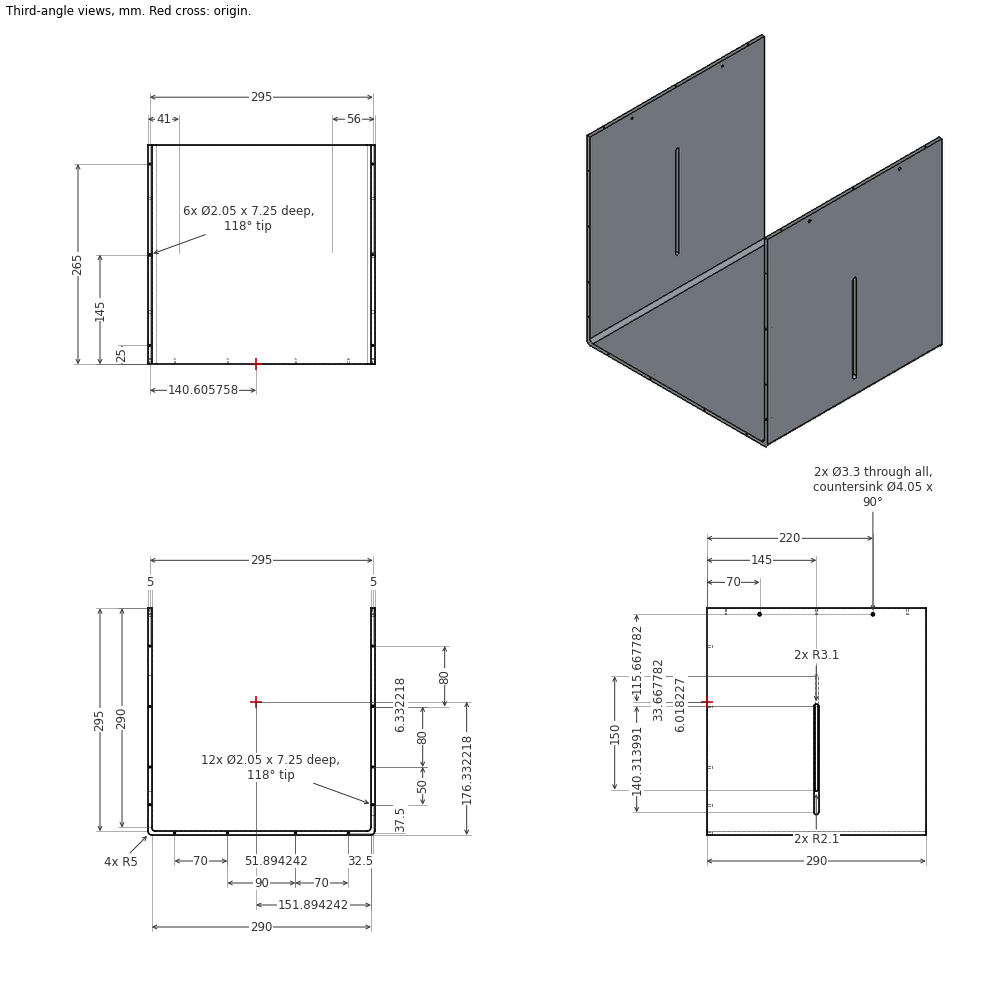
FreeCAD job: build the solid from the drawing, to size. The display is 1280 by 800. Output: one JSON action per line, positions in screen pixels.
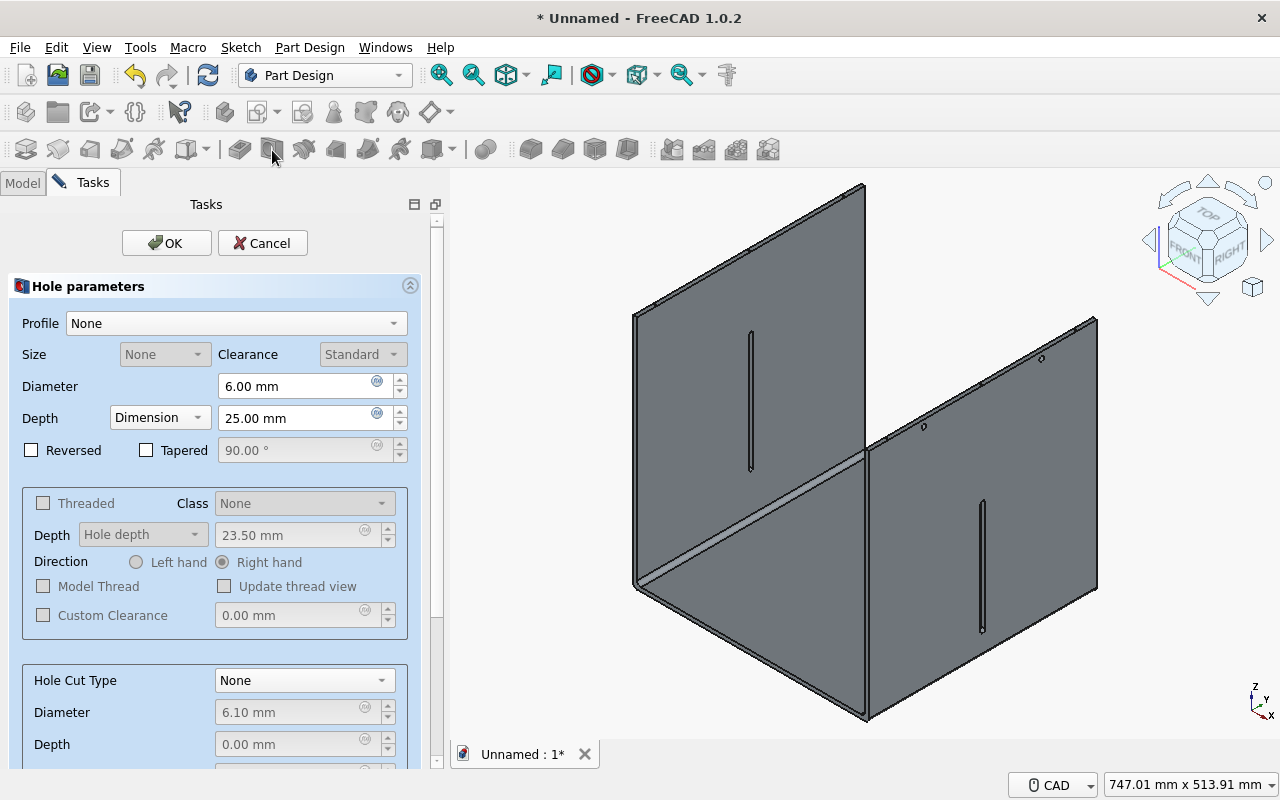
{"action": "triple_click", "coordinate": [305, 386]}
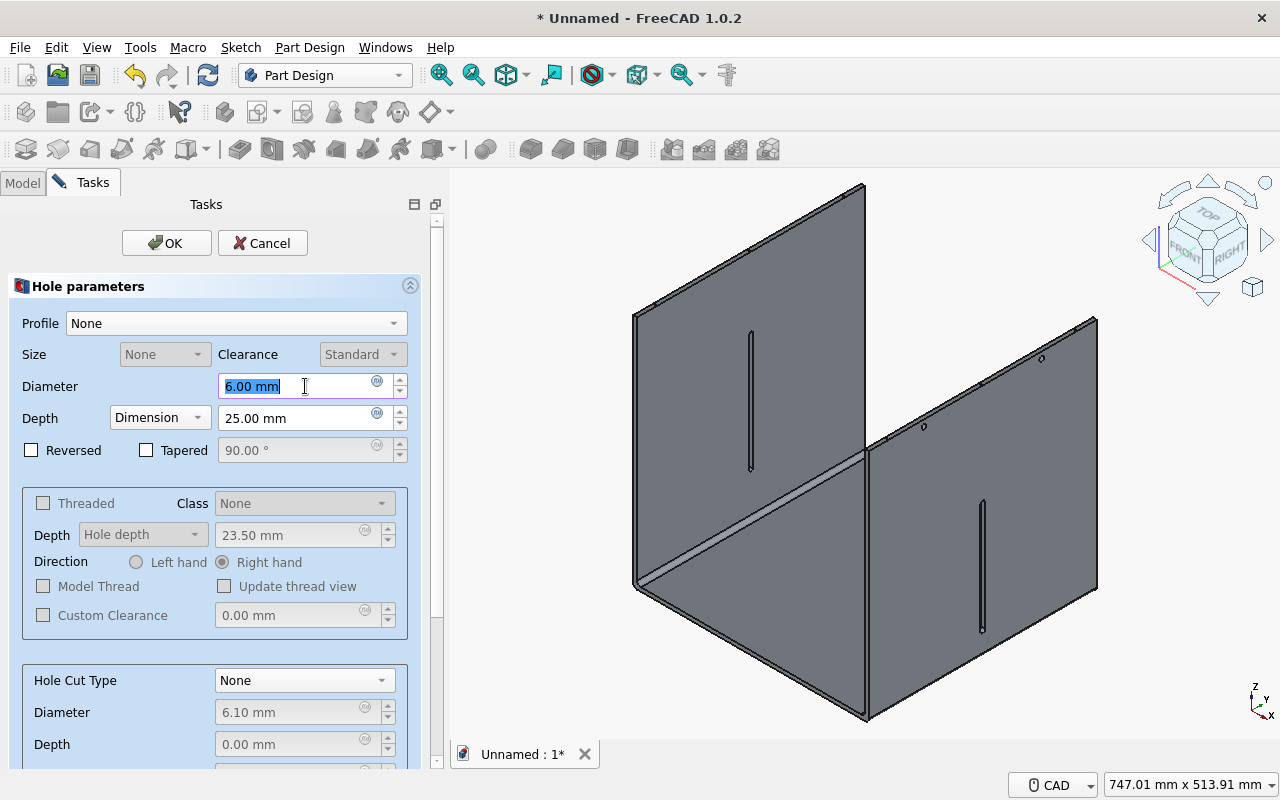
{"action": "type", "text": "3.3"}
{"action": "key", "text": "Tab"}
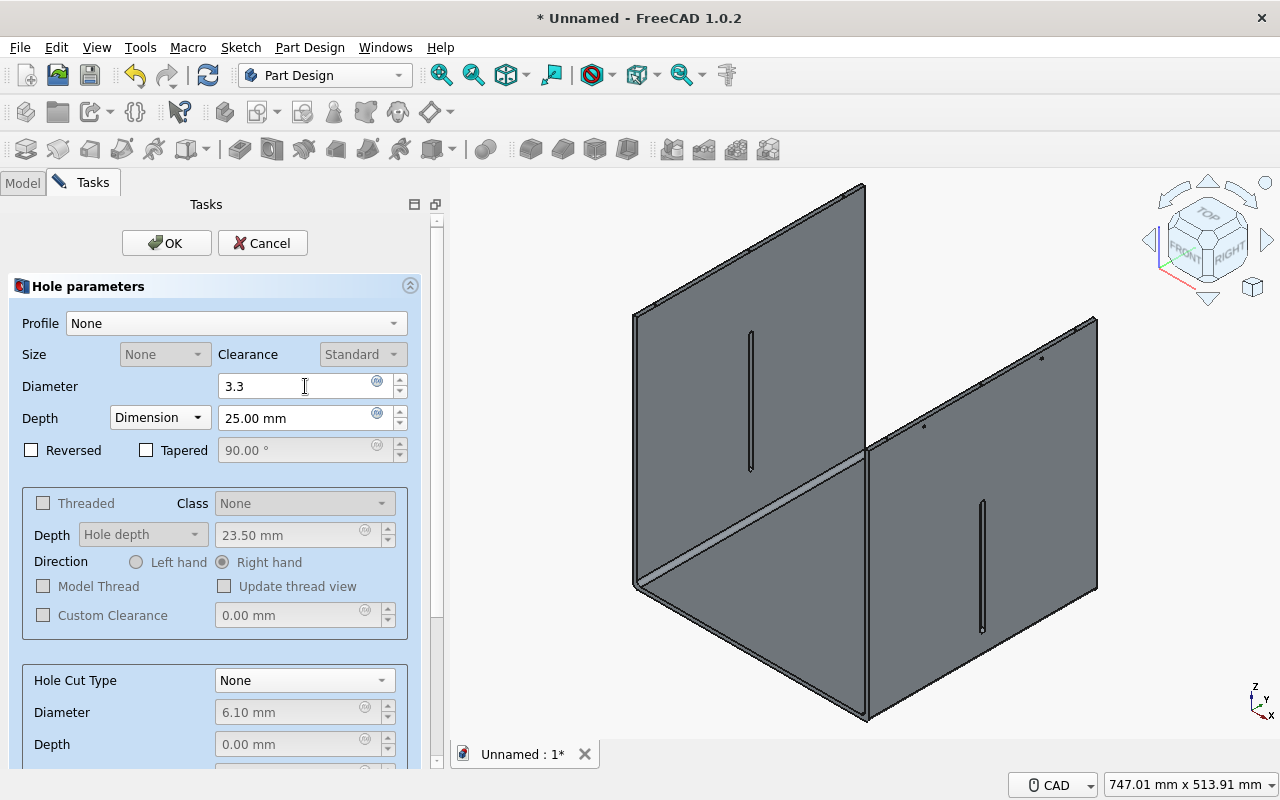
{"action": "left_click", "coordinate": [161, 418]}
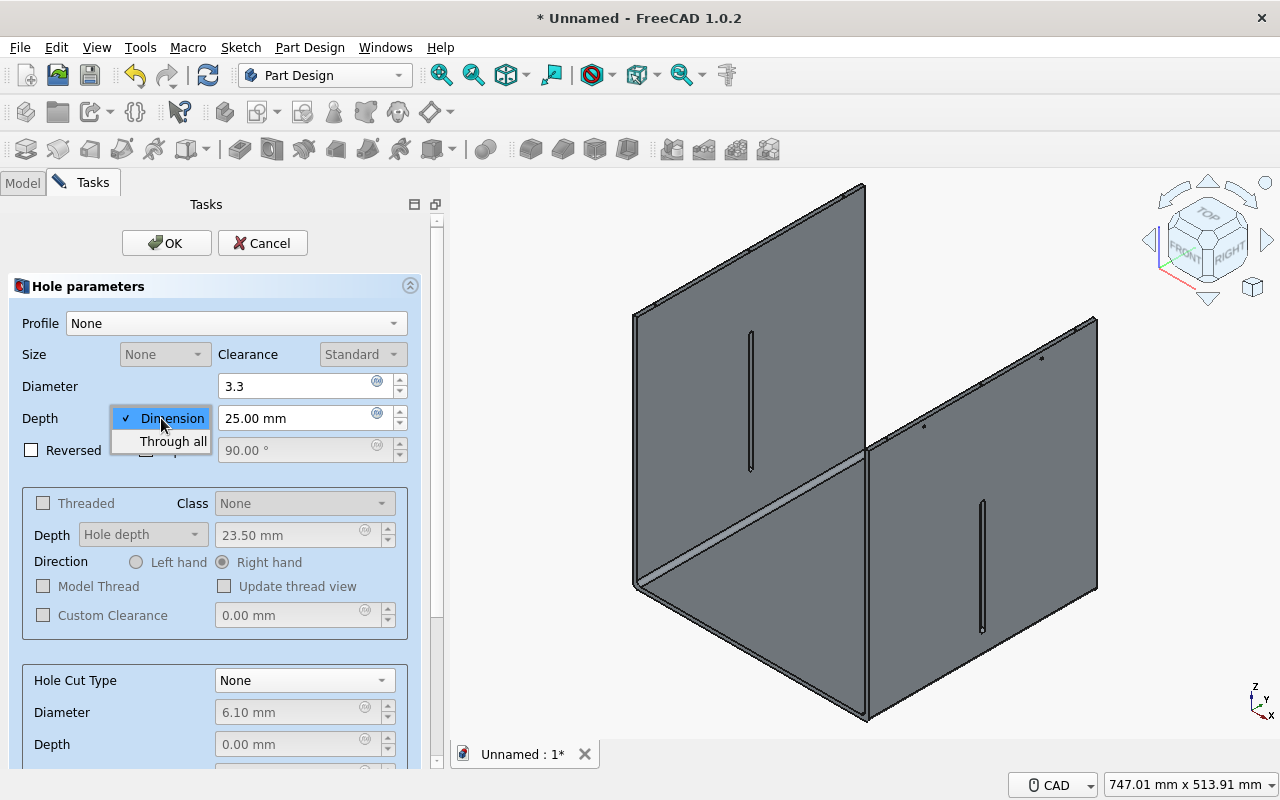
{"action": "left_click", "coordinate": [160, 442]}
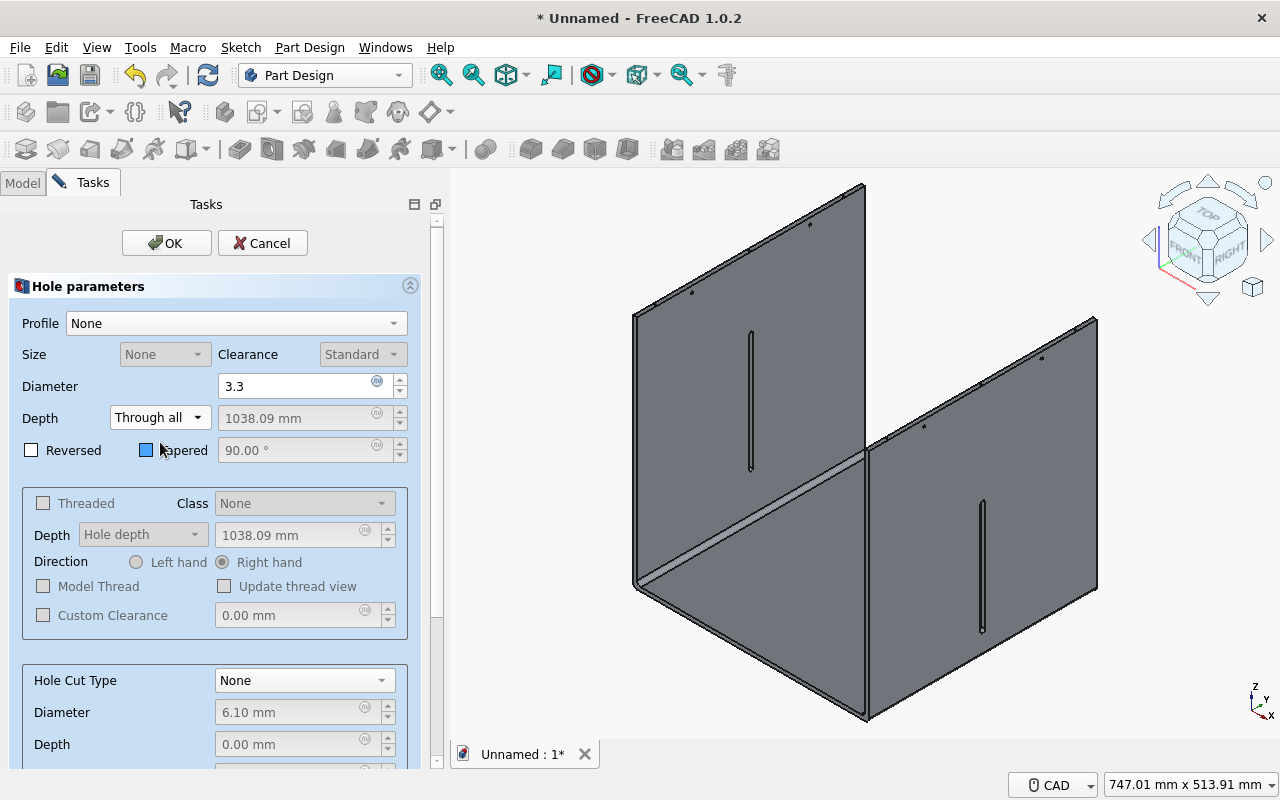
{"action": "left_click", "coordinate": [306, 680]}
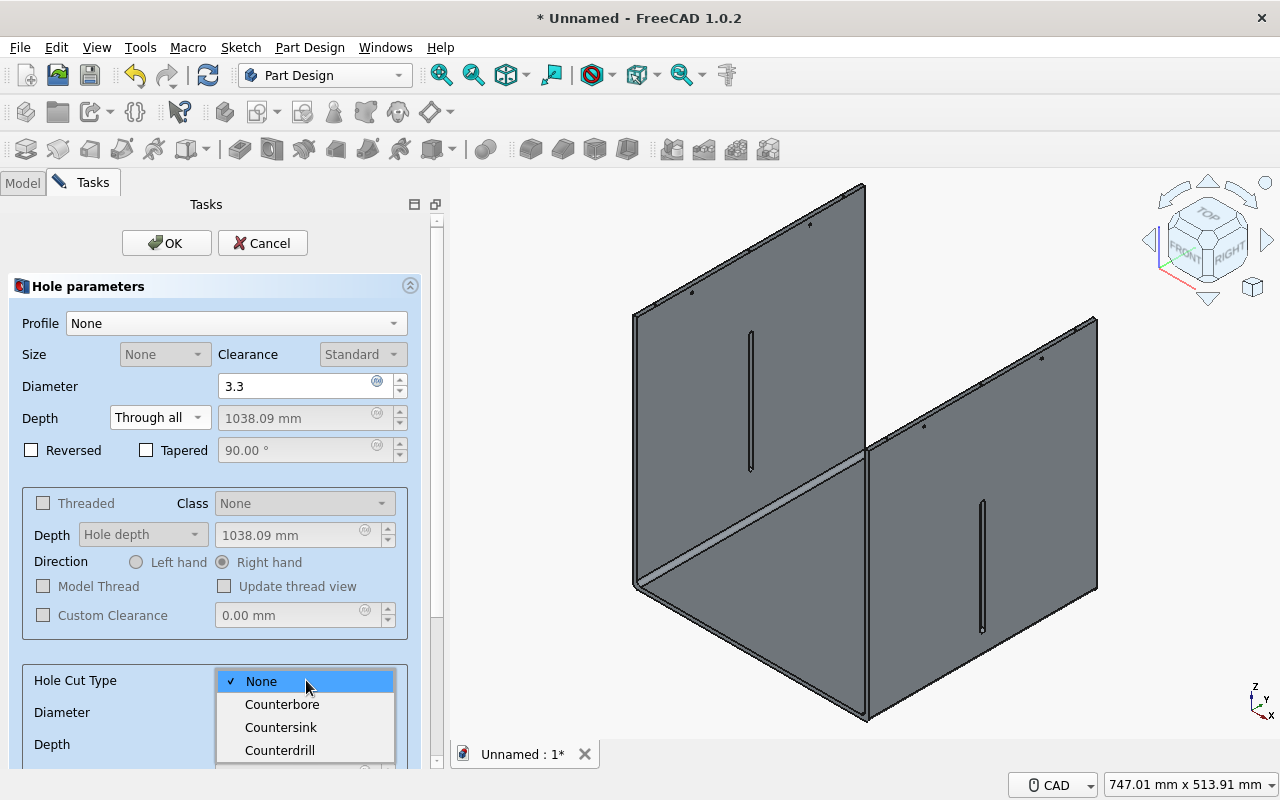
{"action": "left_click", "coordinate": [304, 728]}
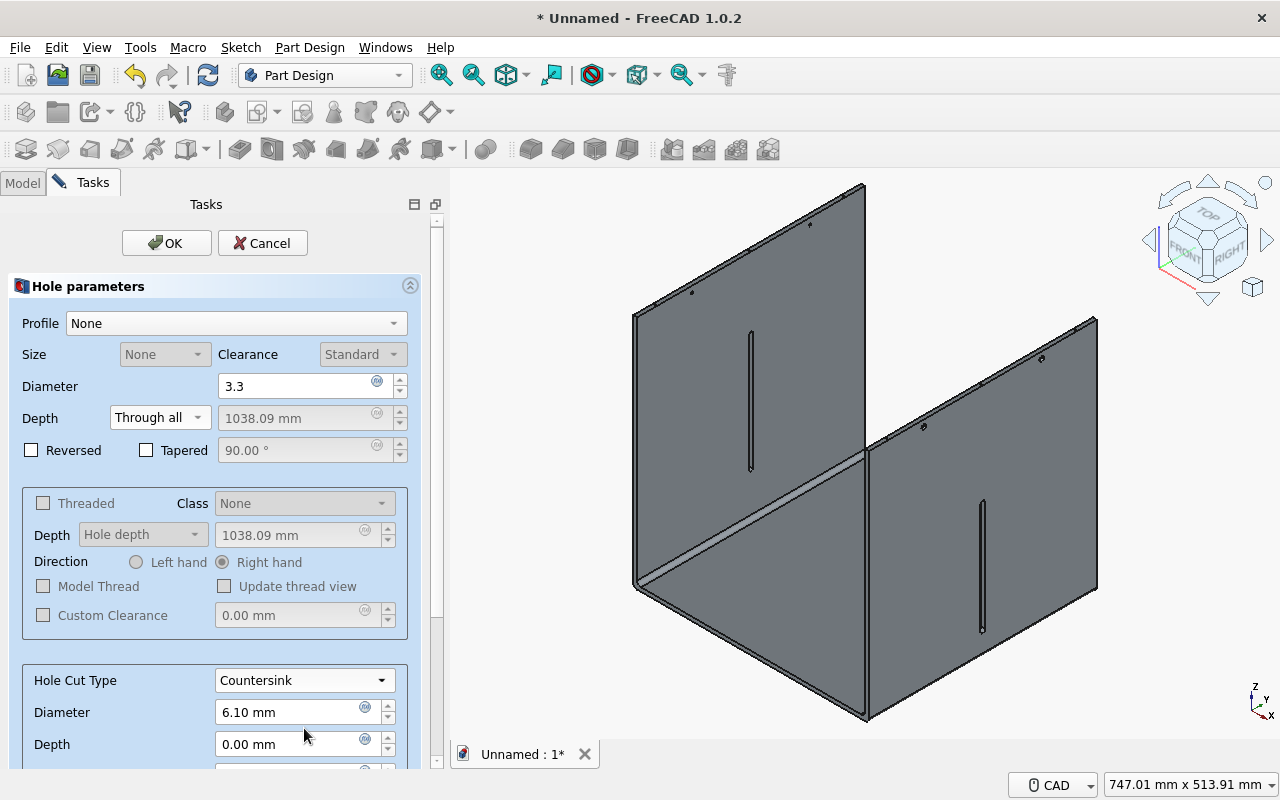
{"action": "triple_click", "coordinate": [298, 712]}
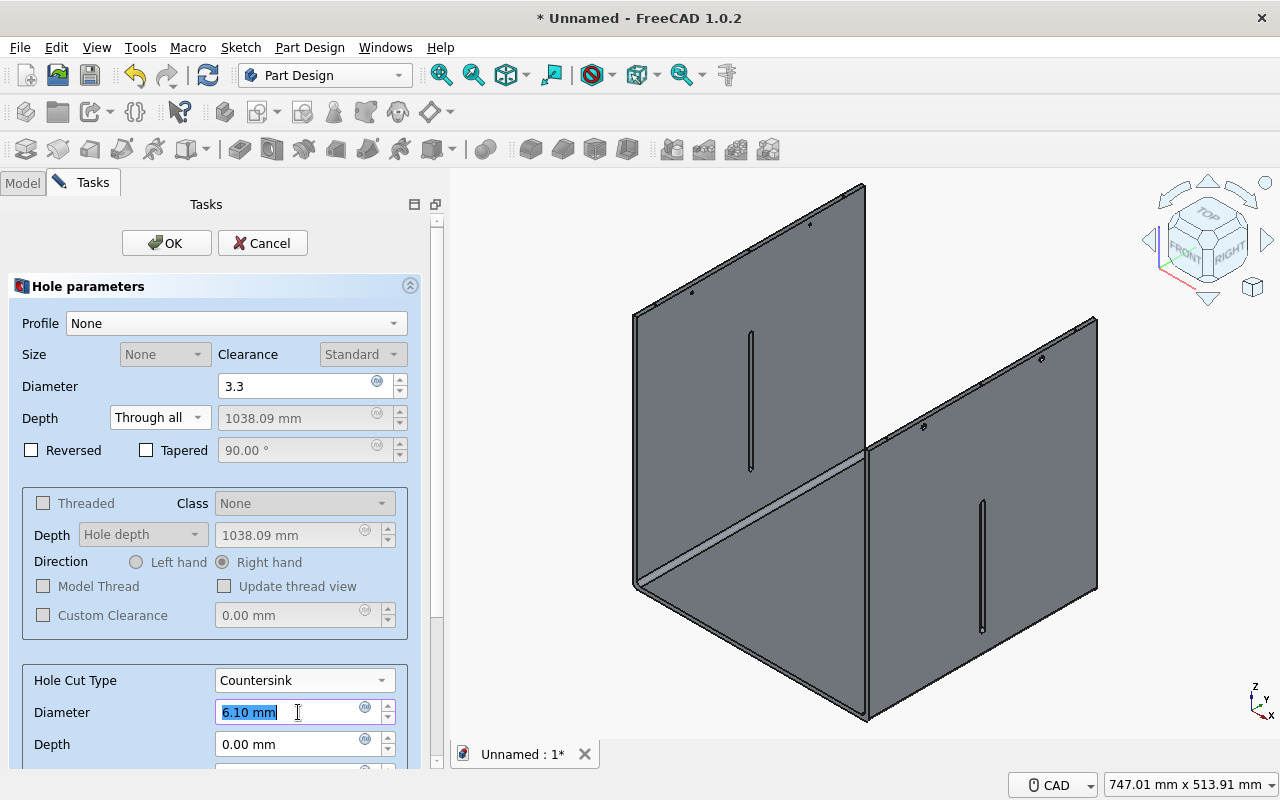
{"action": "type", "text": "4.05"}
{"action": "key", "text": "Tab"}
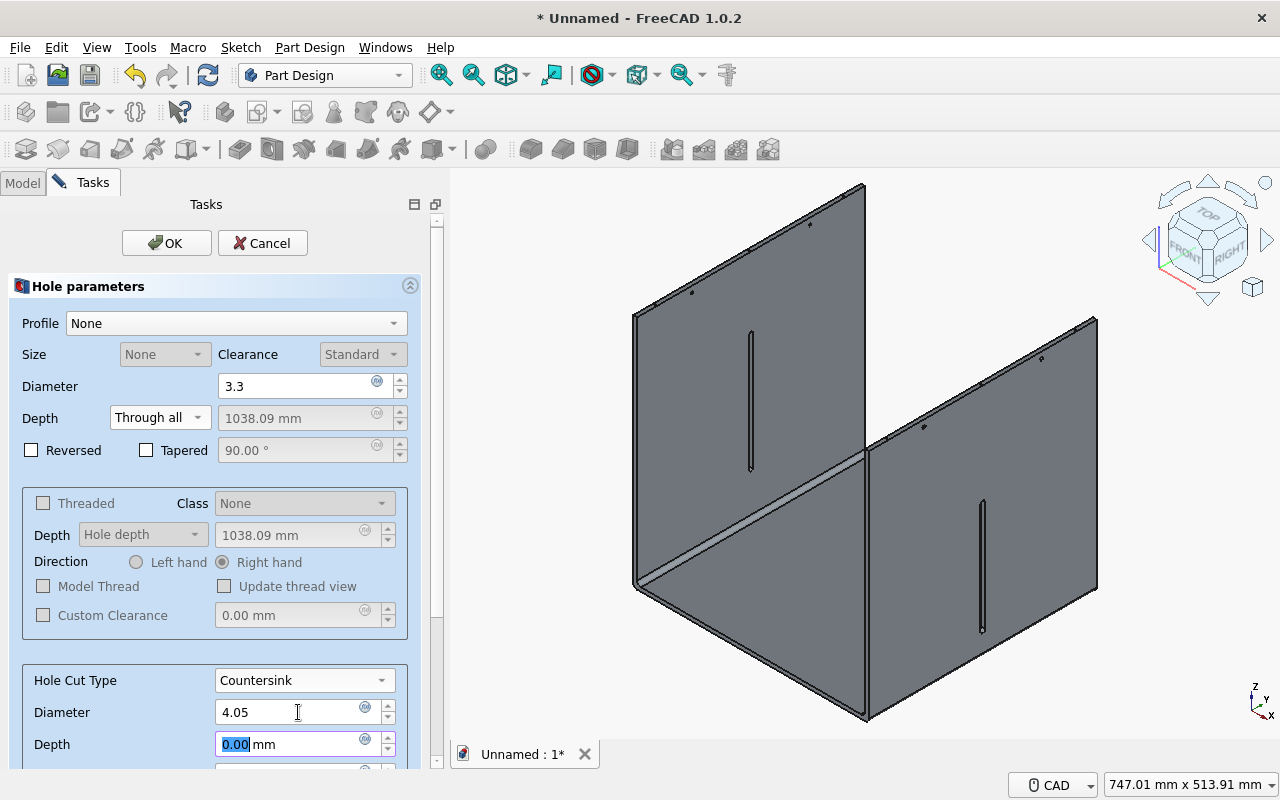
{"action": "left_click", "coordinate": [167, 243]}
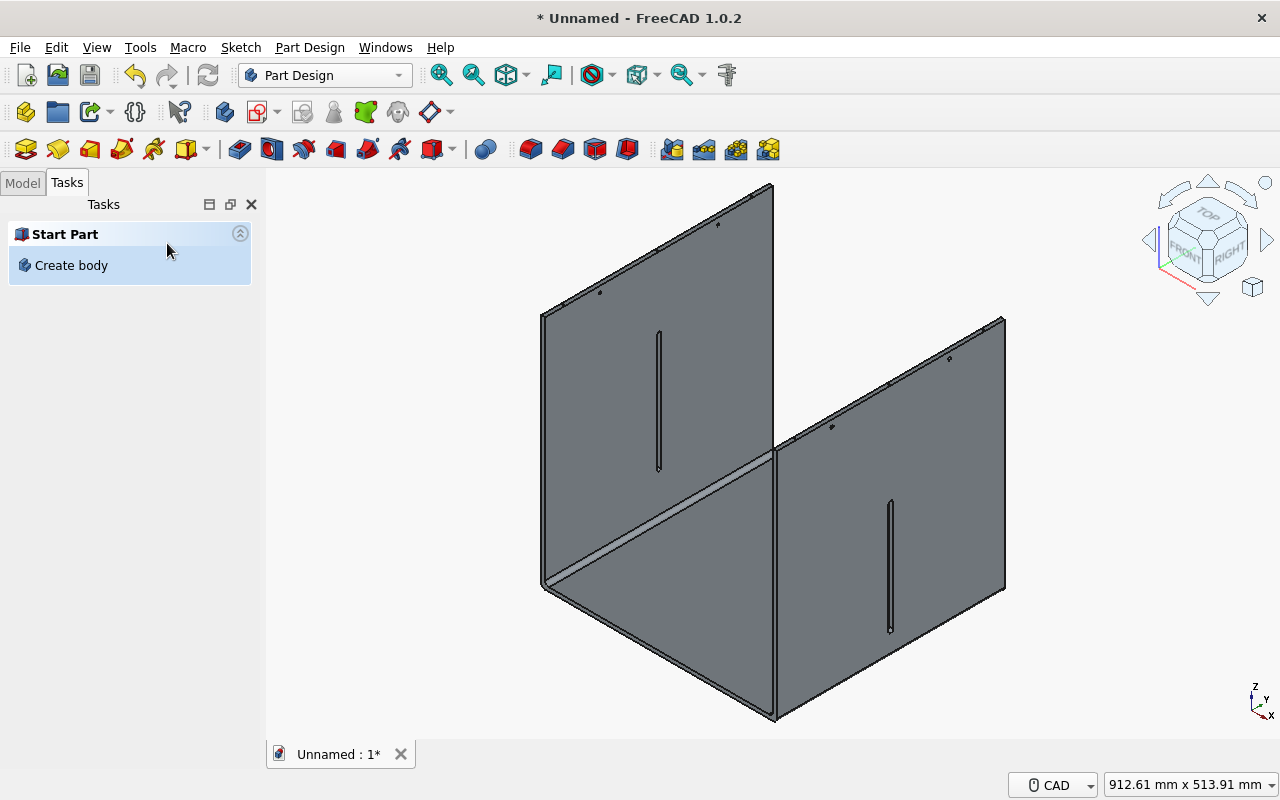
{"action": "left_click", "coordinate": [258, 112]}